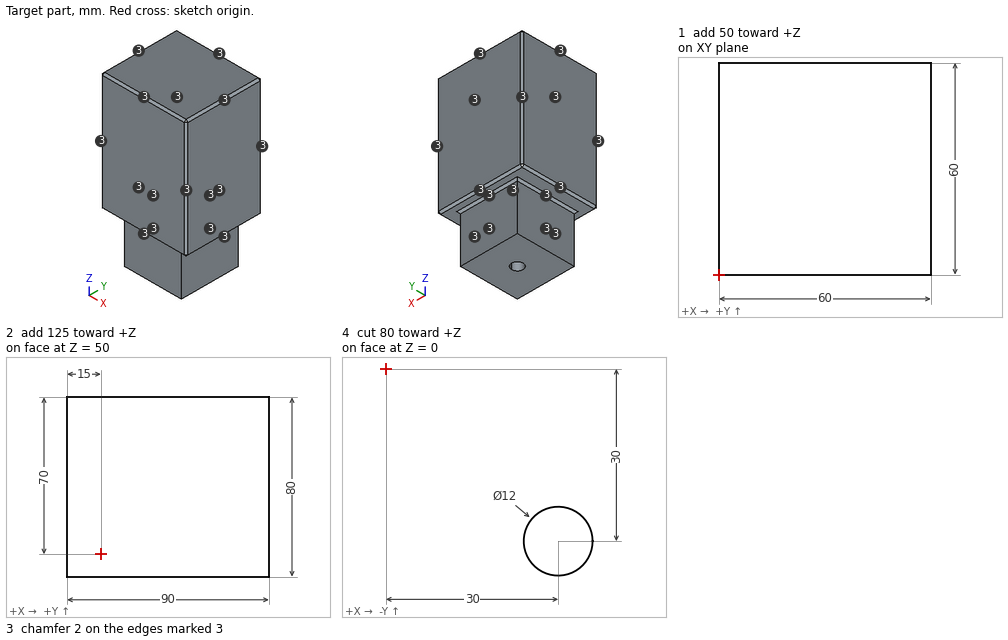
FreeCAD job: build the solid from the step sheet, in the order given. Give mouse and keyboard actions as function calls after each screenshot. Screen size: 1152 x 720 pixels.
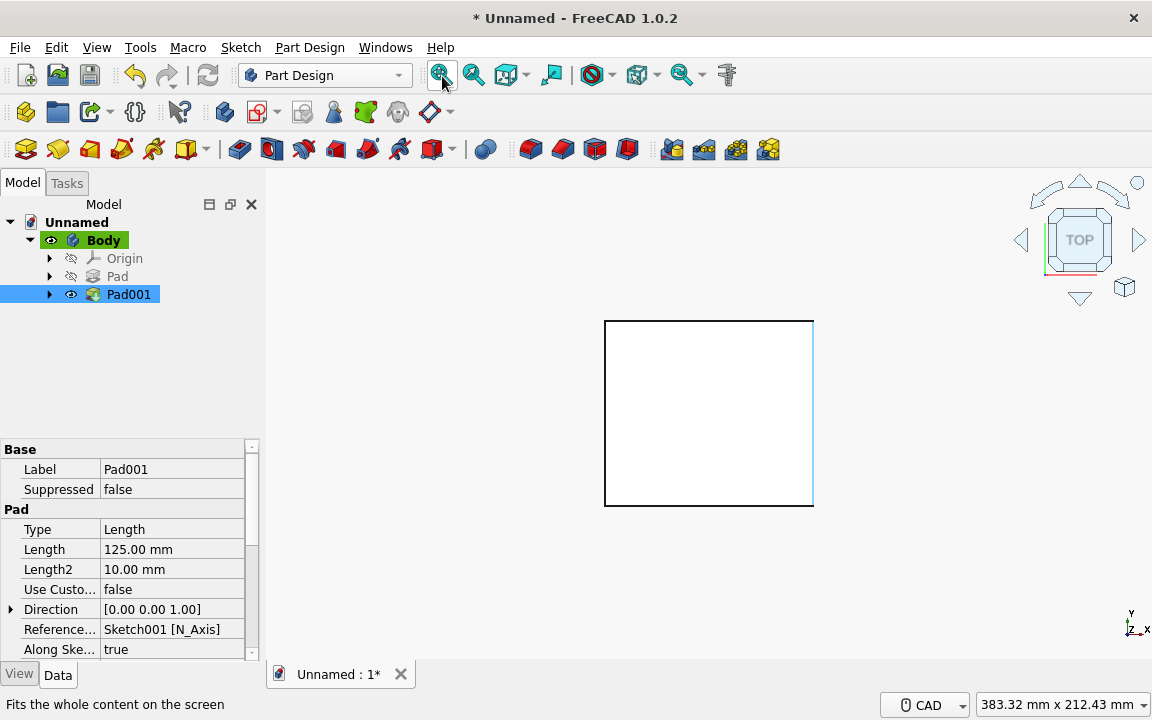
key(v)
key(f)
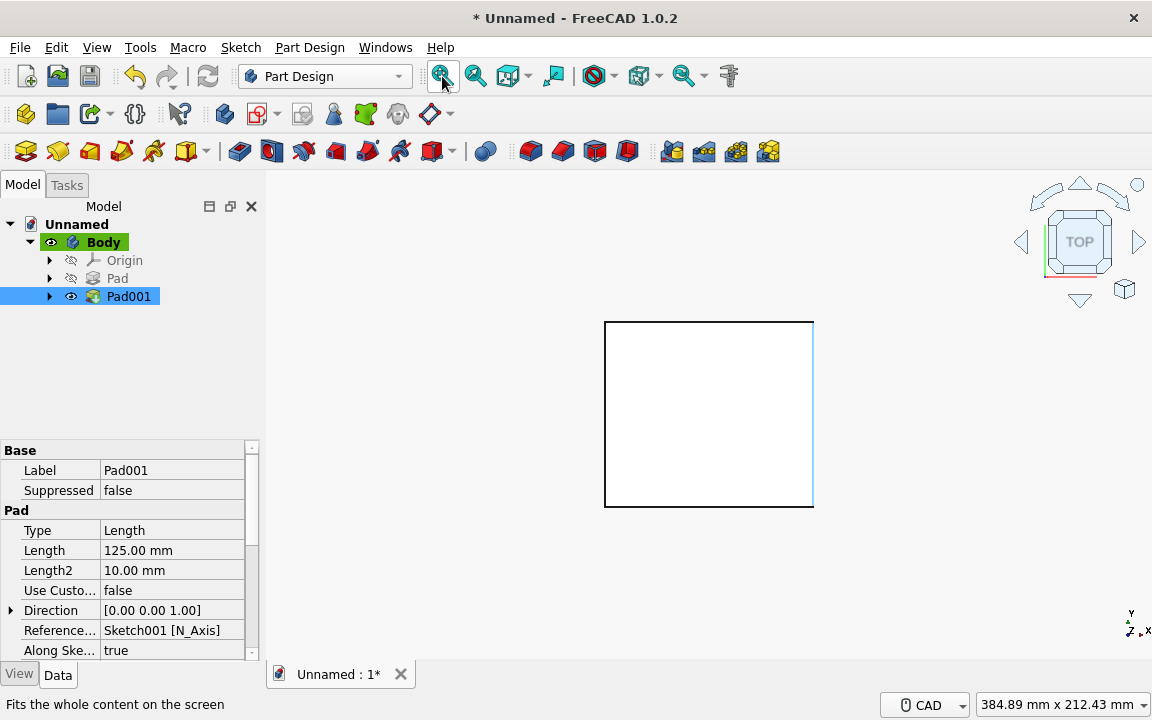
click(605, 413, ctrl)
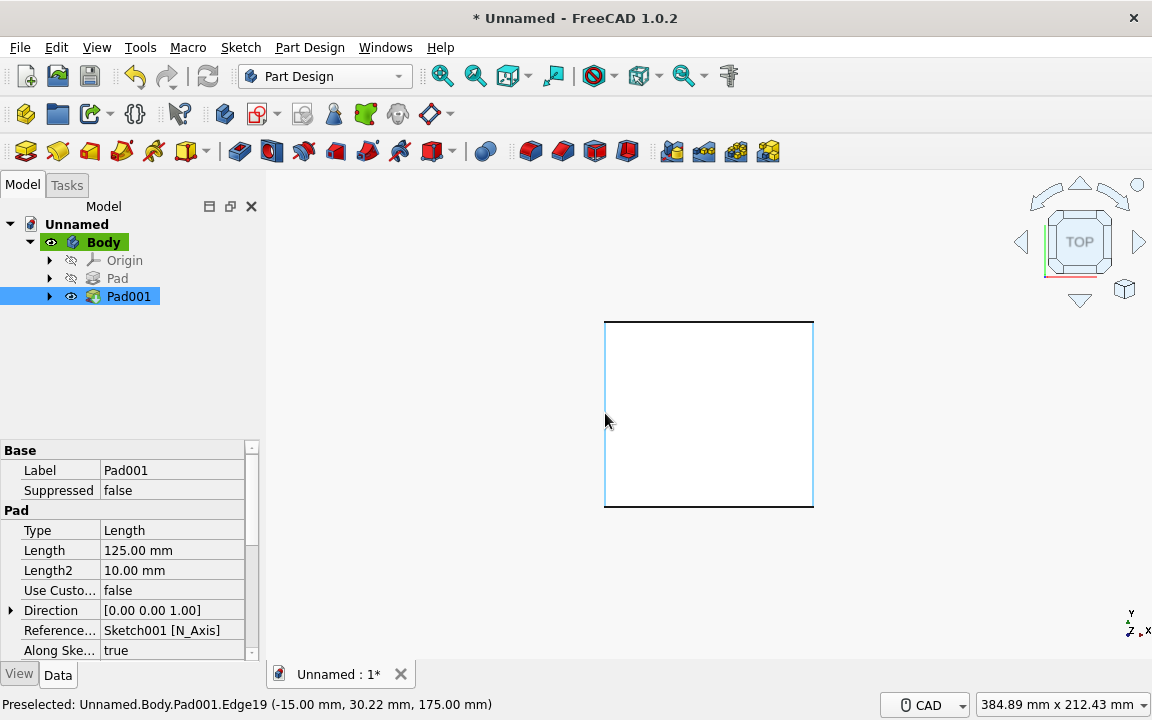
key(1)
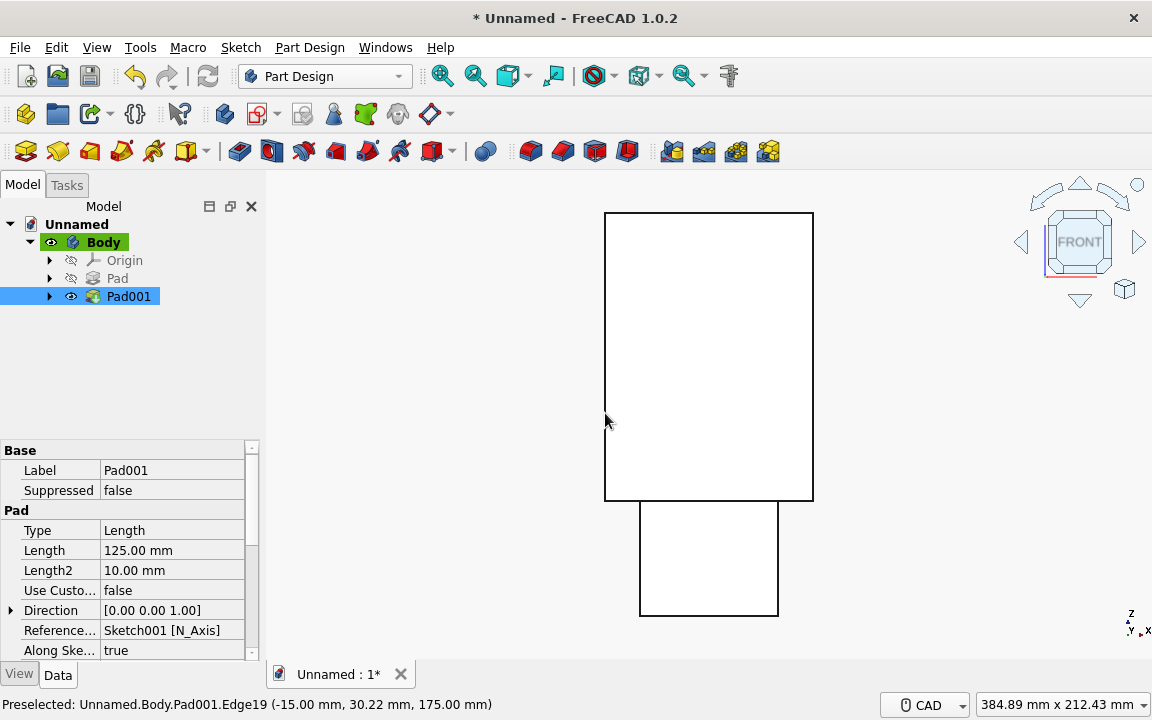
key(3)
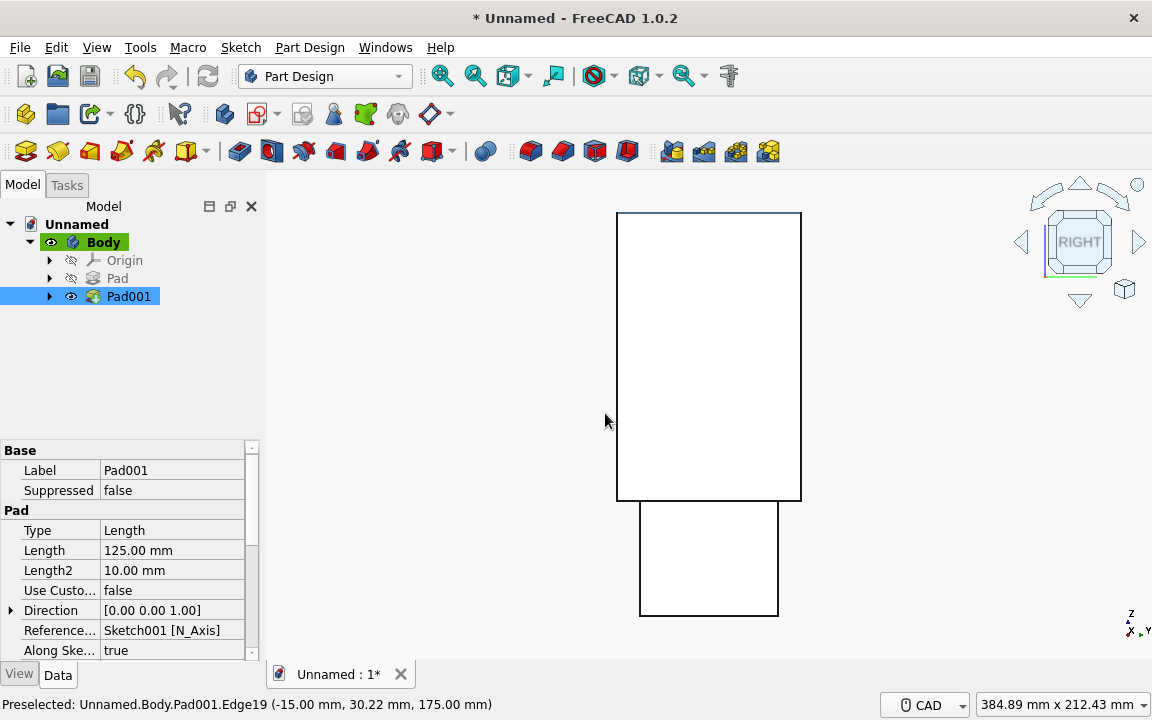
key(5)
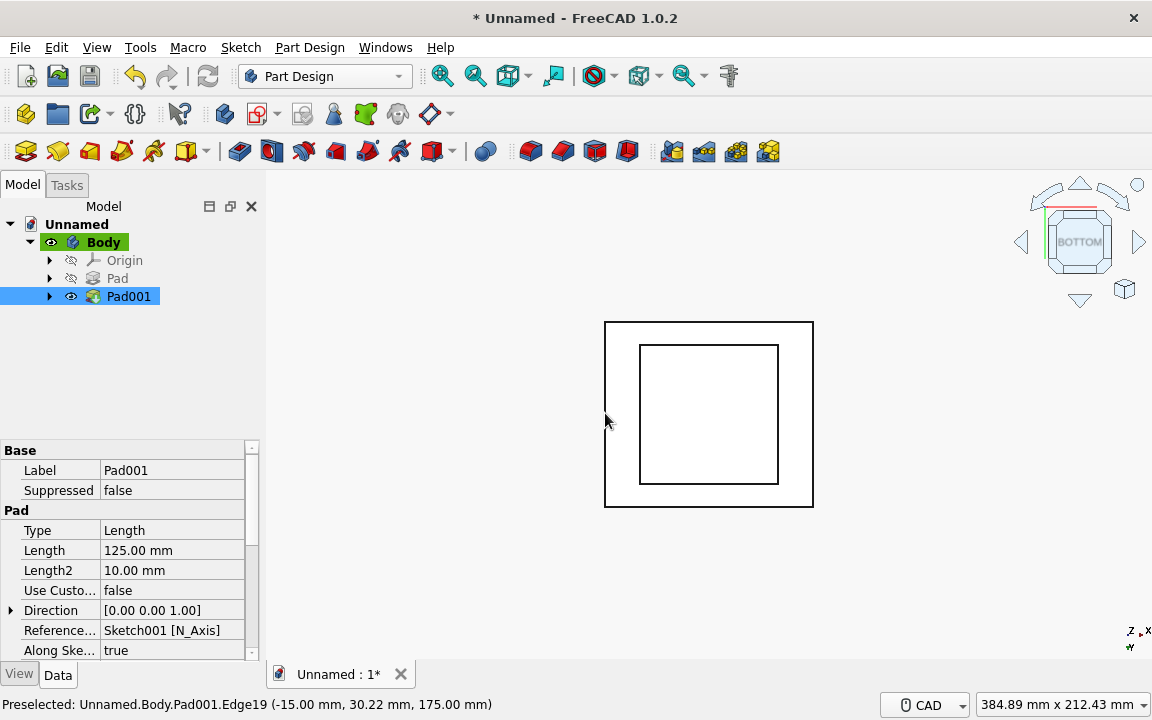
key(v)
key(f)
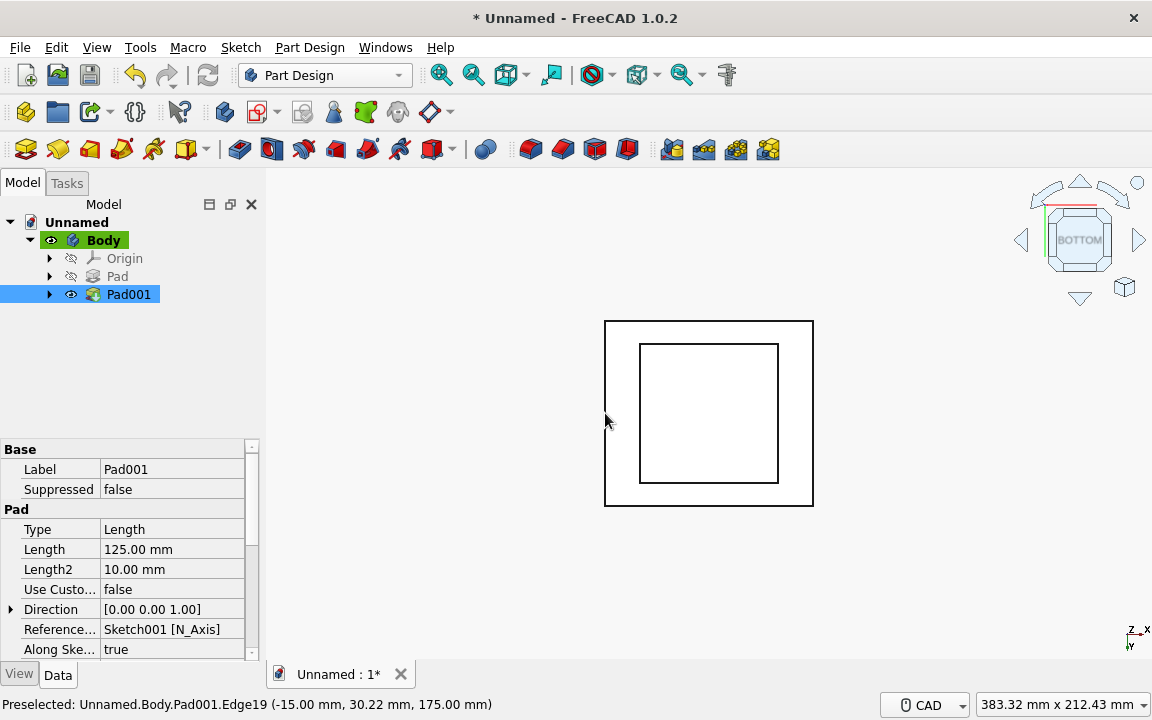
click(798, 465, ctrl)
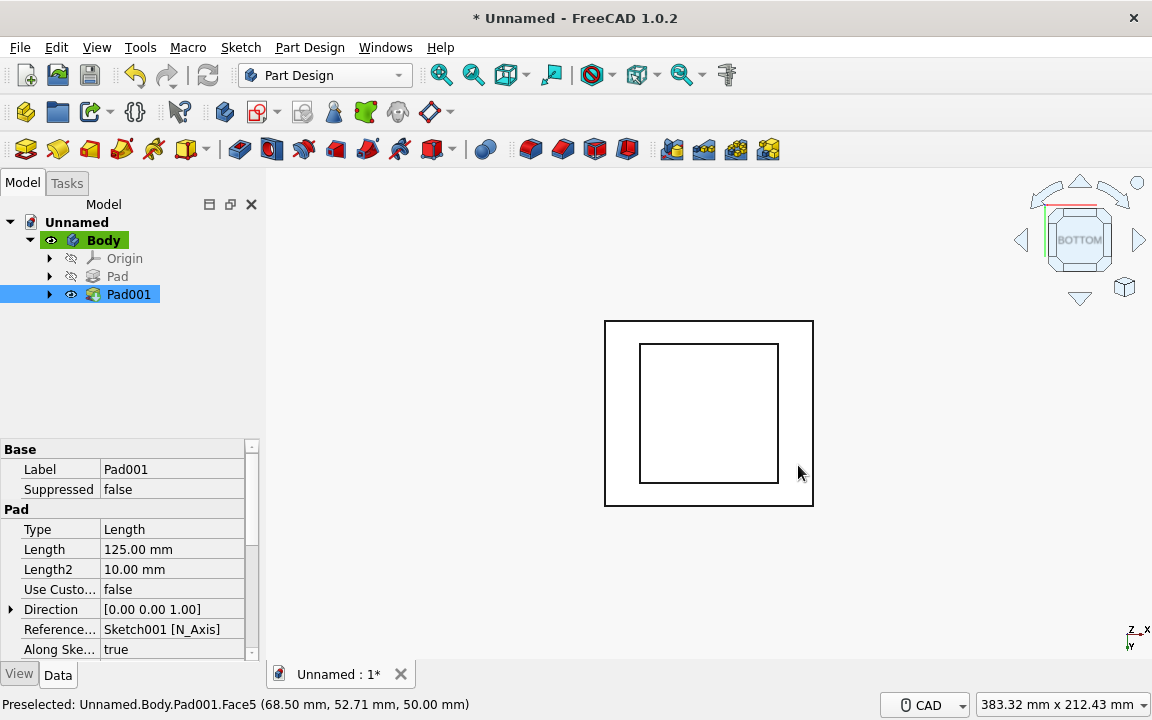
key(4)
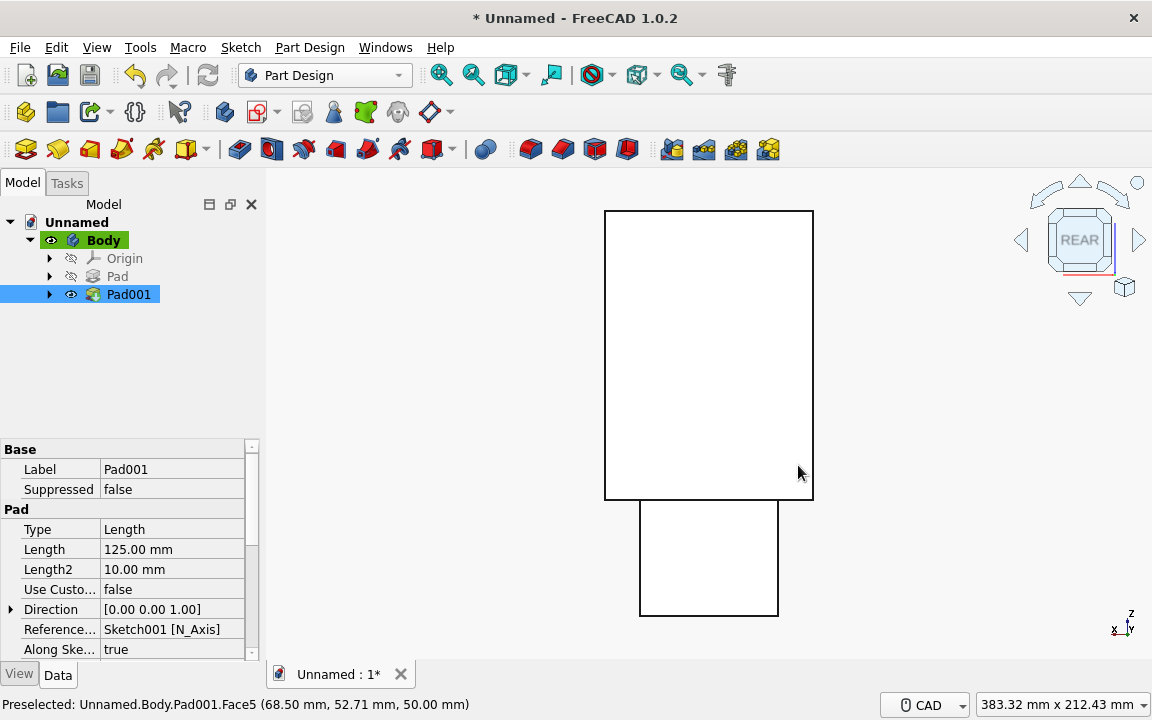
click(709, 355, ctrl)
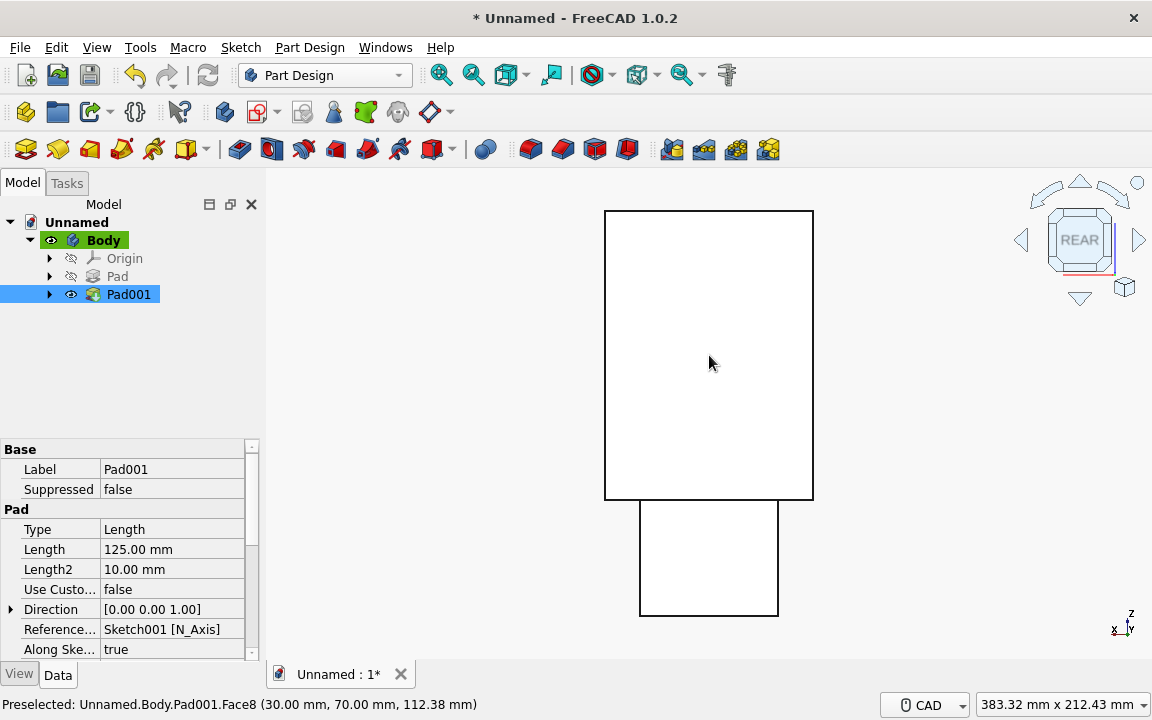
click(564, 150)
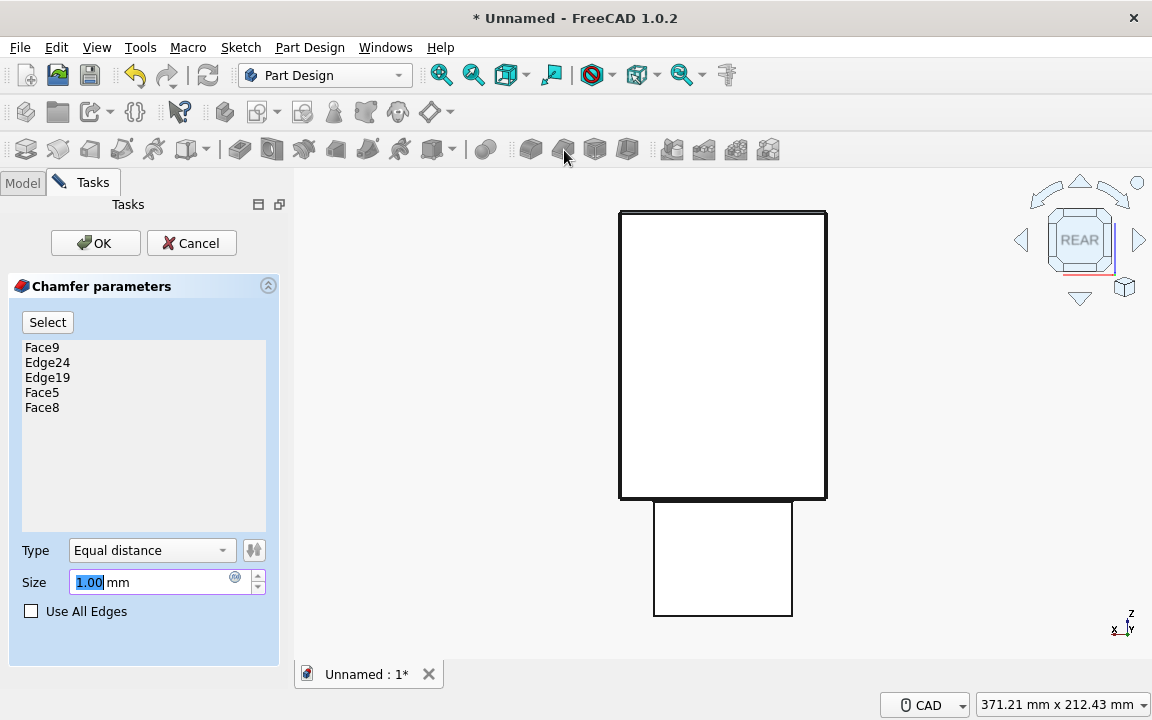
text(2)
key(Tab)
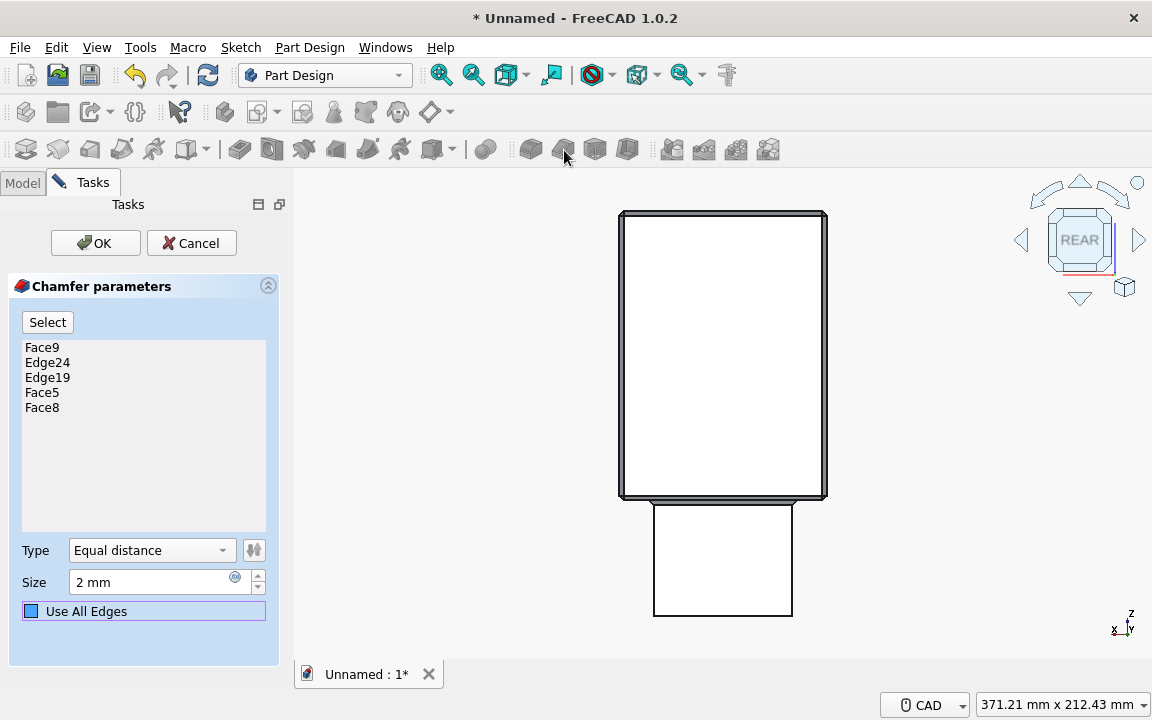
click(96, 243)